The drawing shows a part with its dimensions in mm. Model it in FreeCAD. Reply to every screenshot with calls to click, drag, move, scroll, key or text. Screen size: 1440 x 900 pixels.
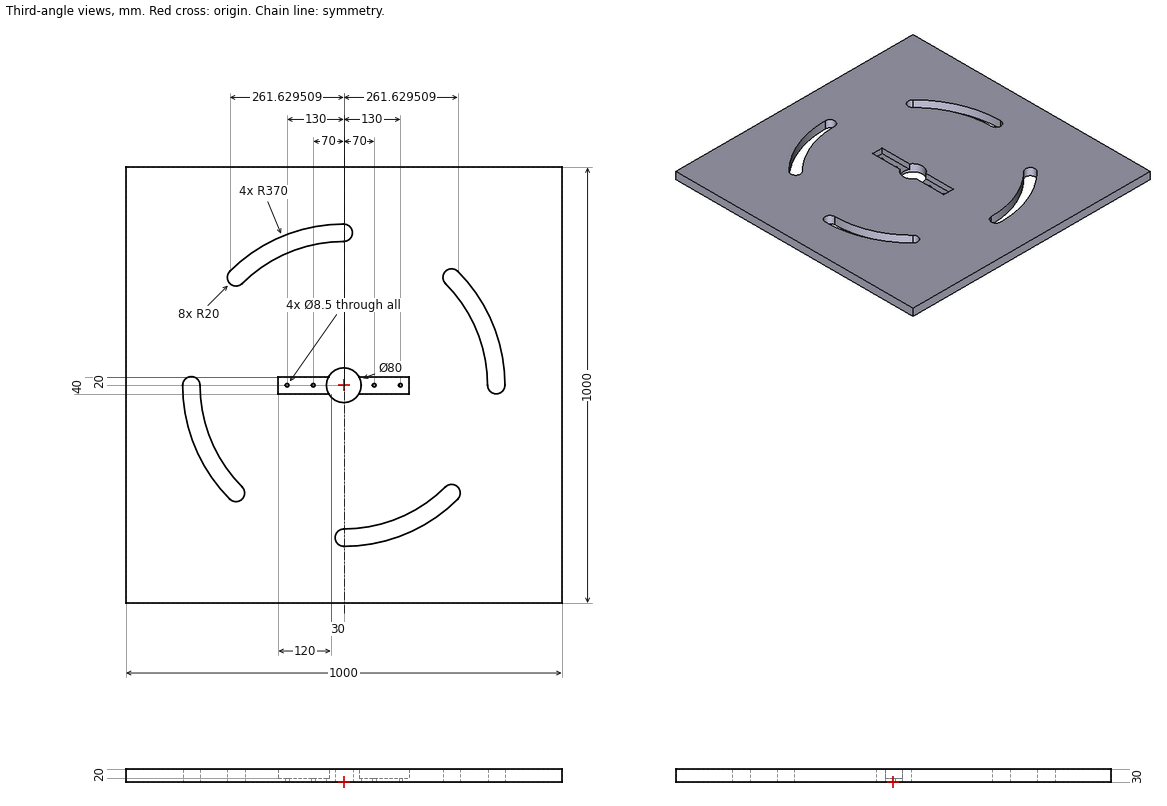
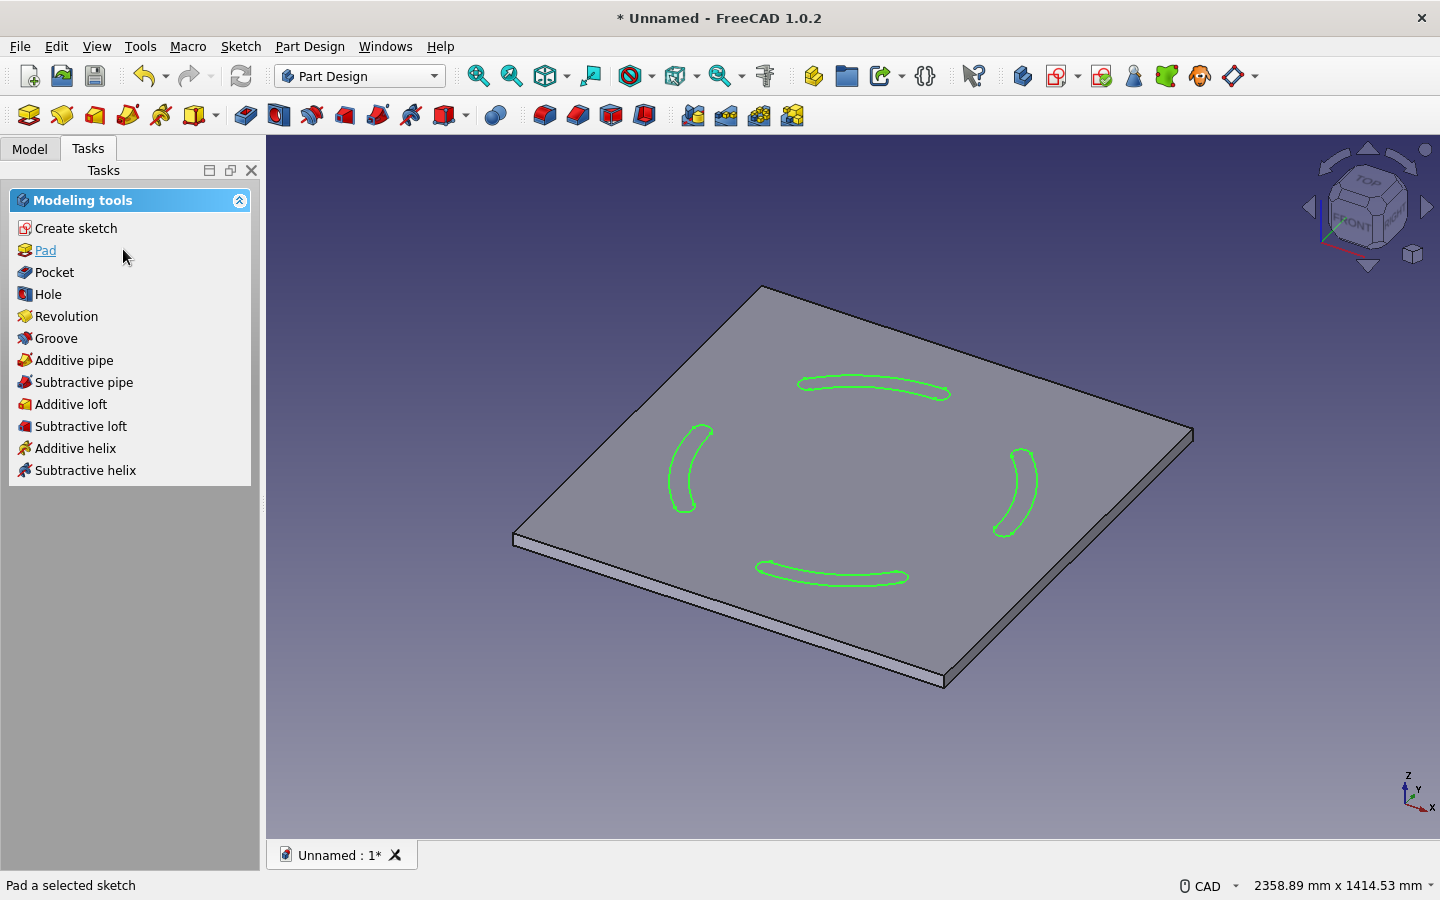
click(246, 116)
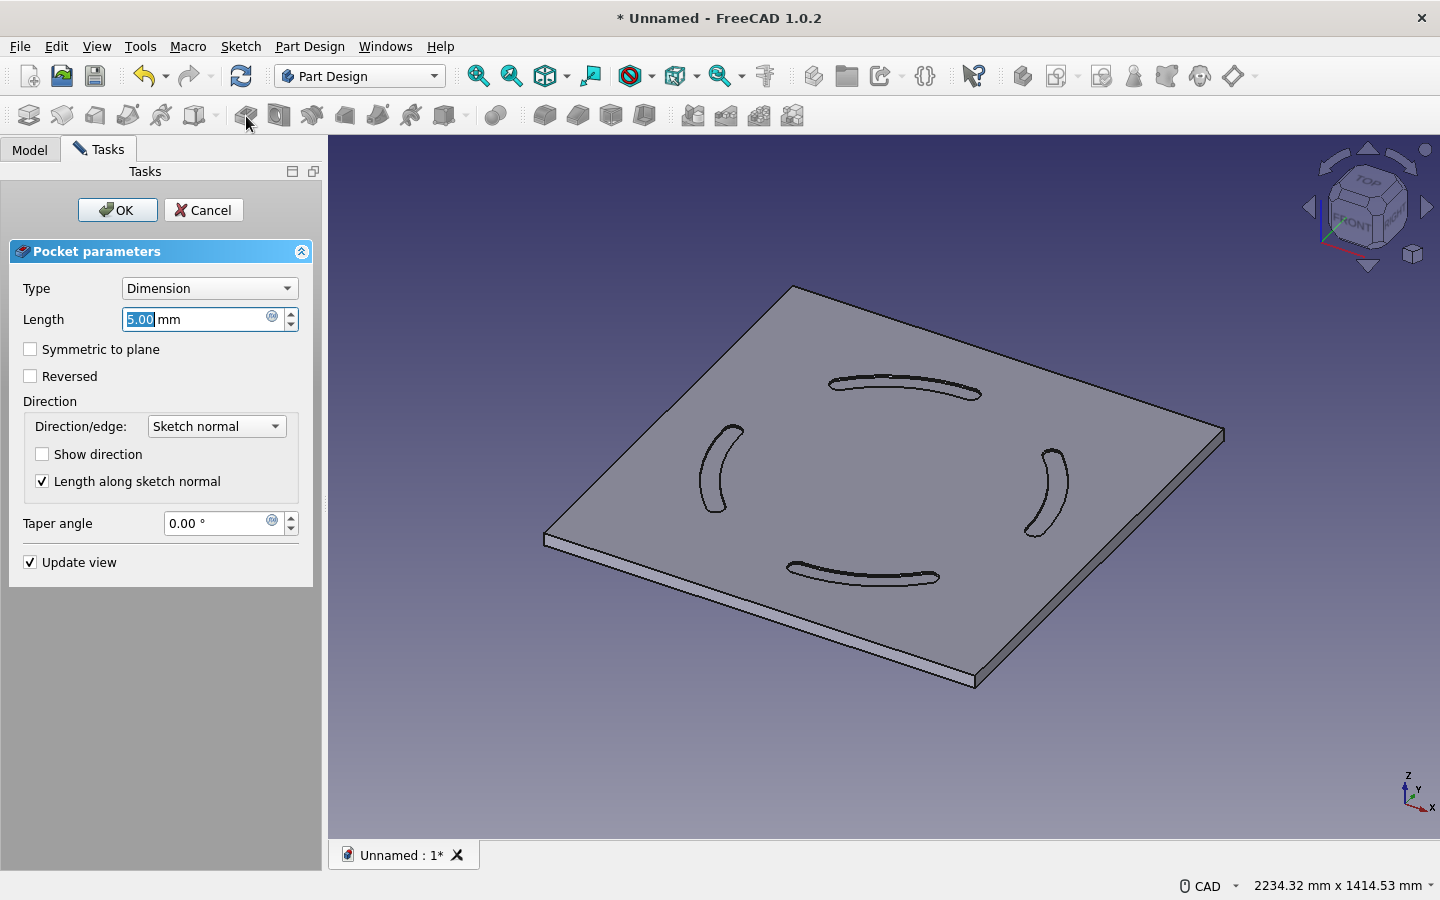
click(210, 288)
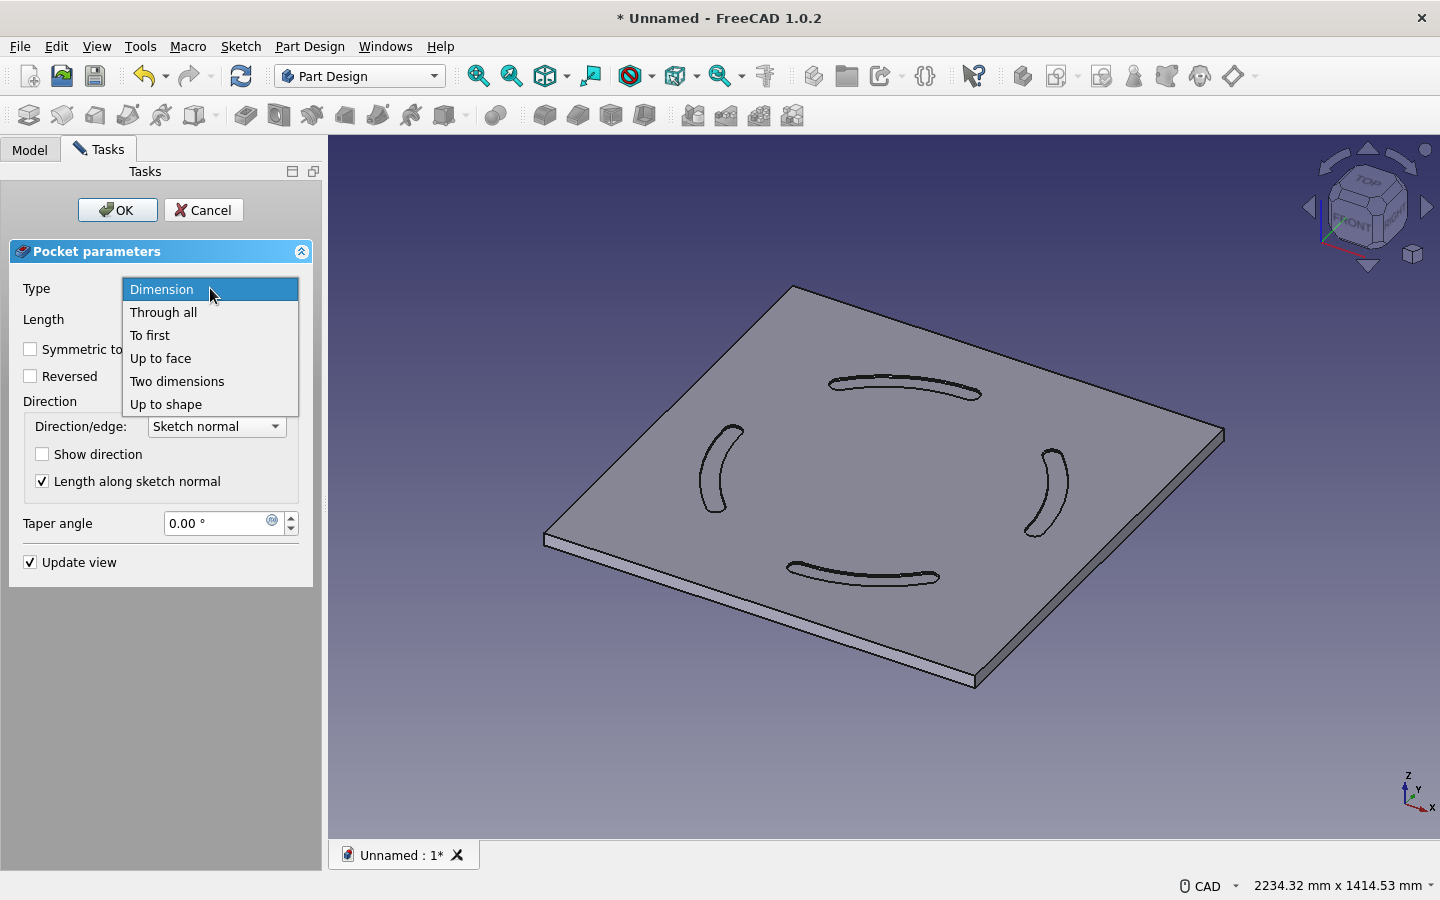
click(208, 312)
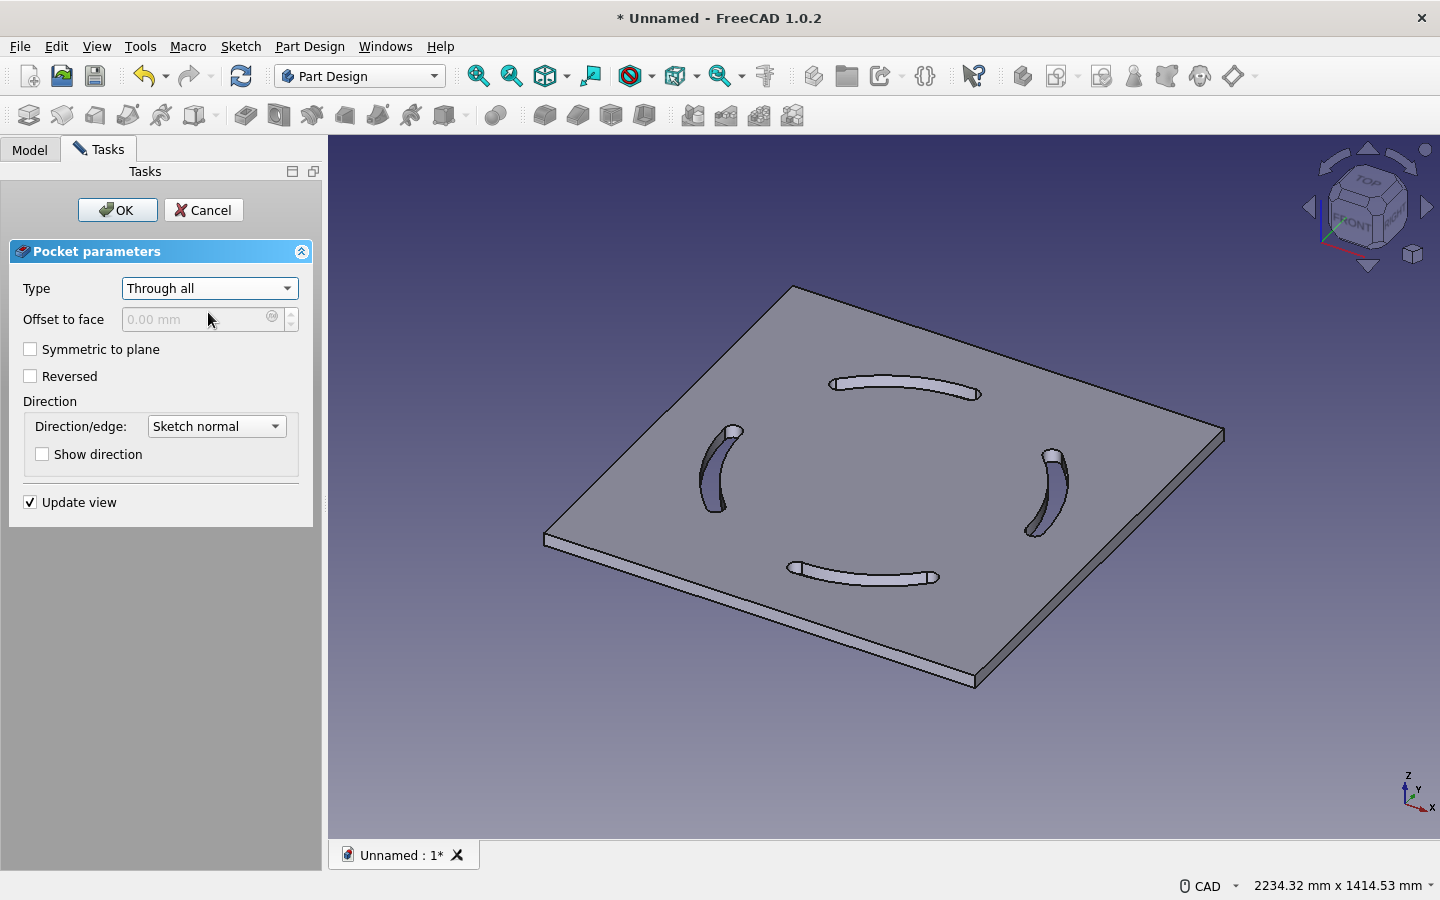
click(118, 210)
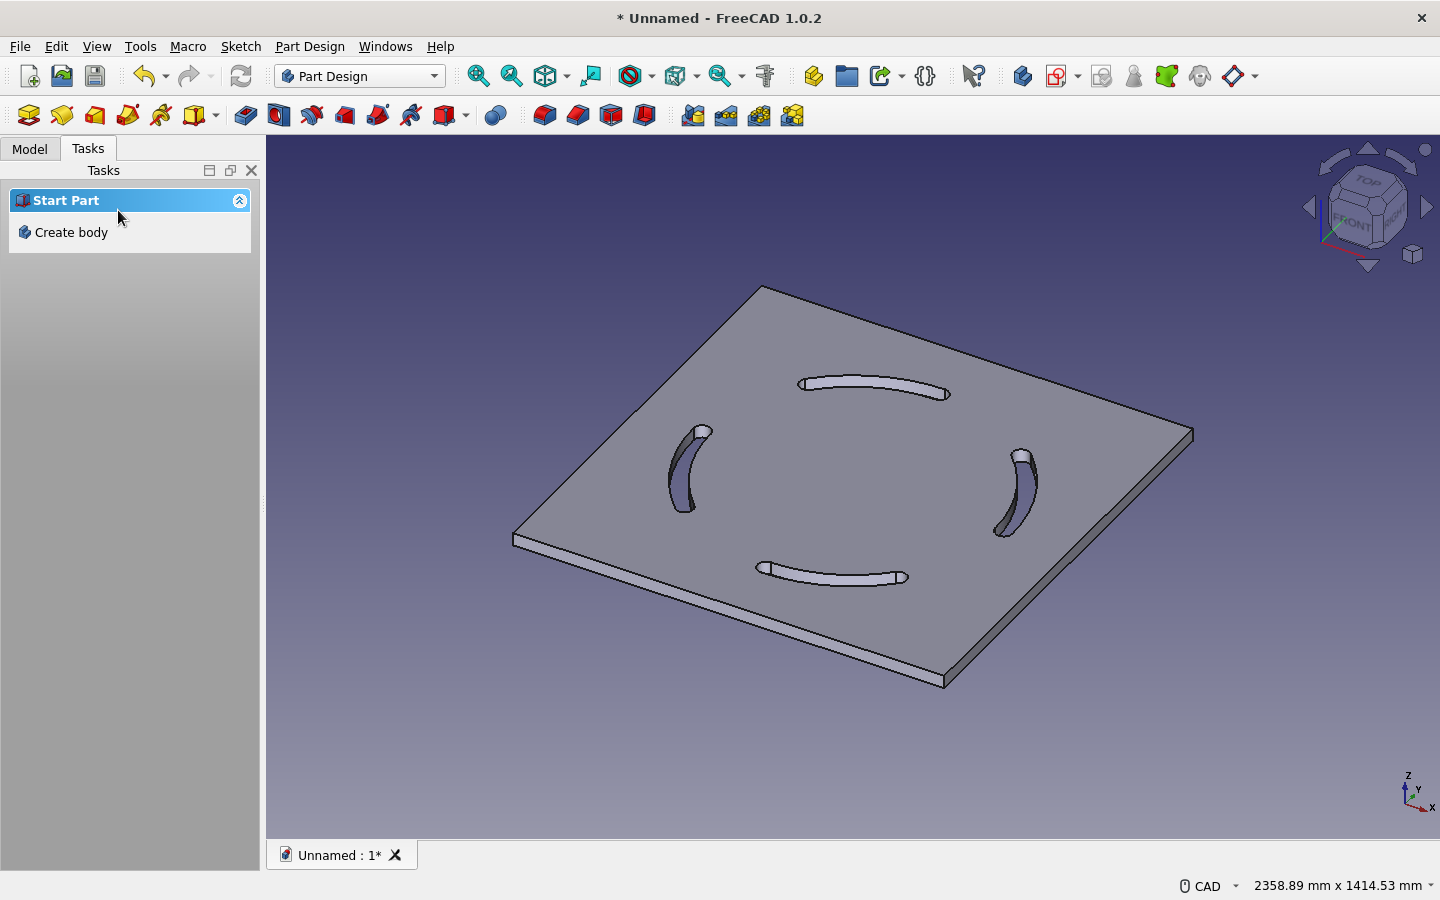
click(853, 480)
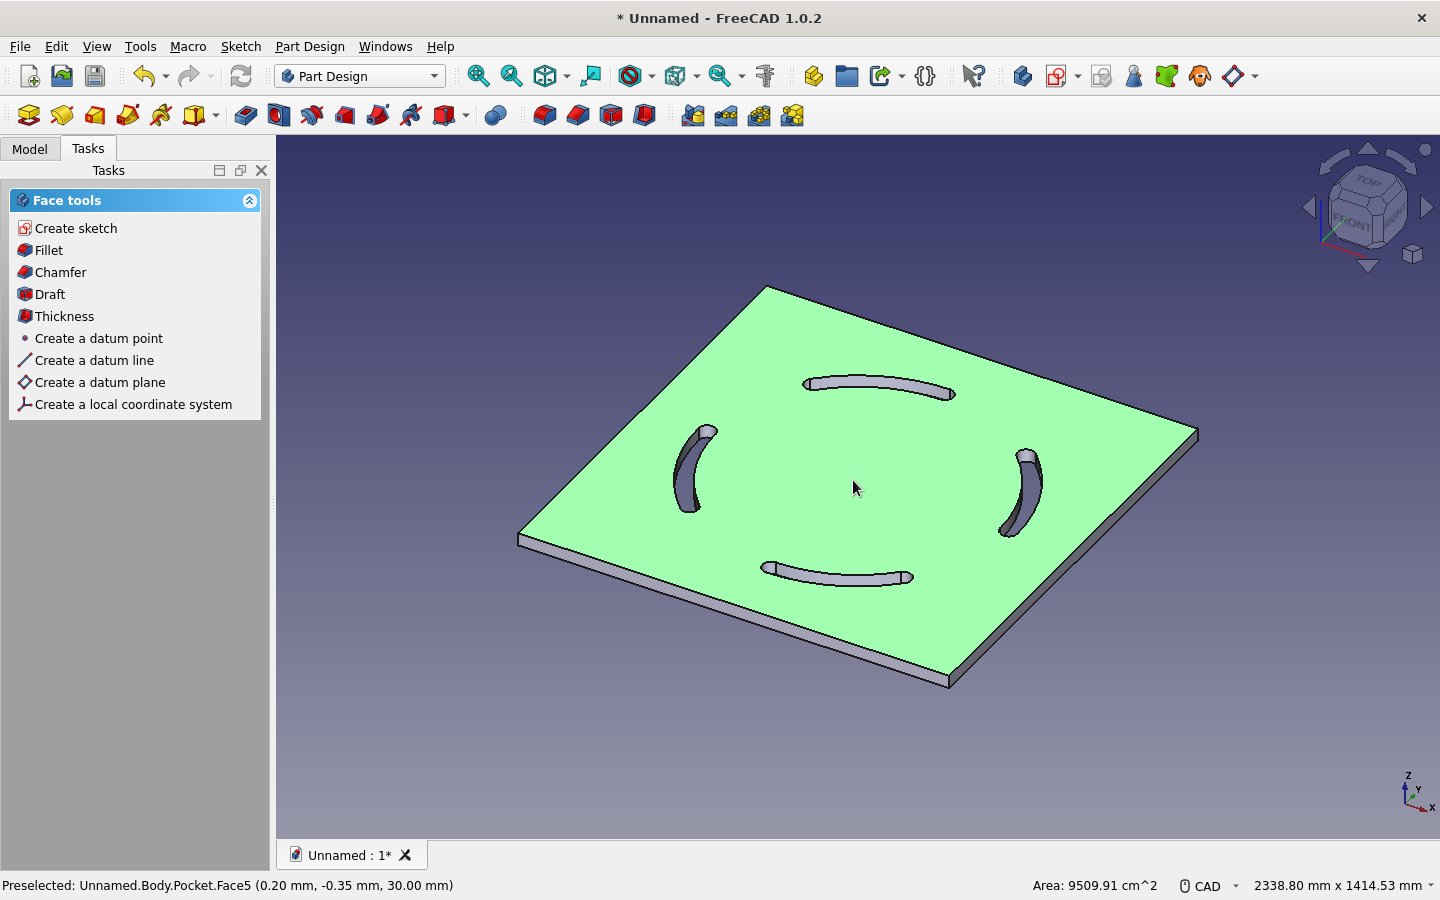
click(1056, 76)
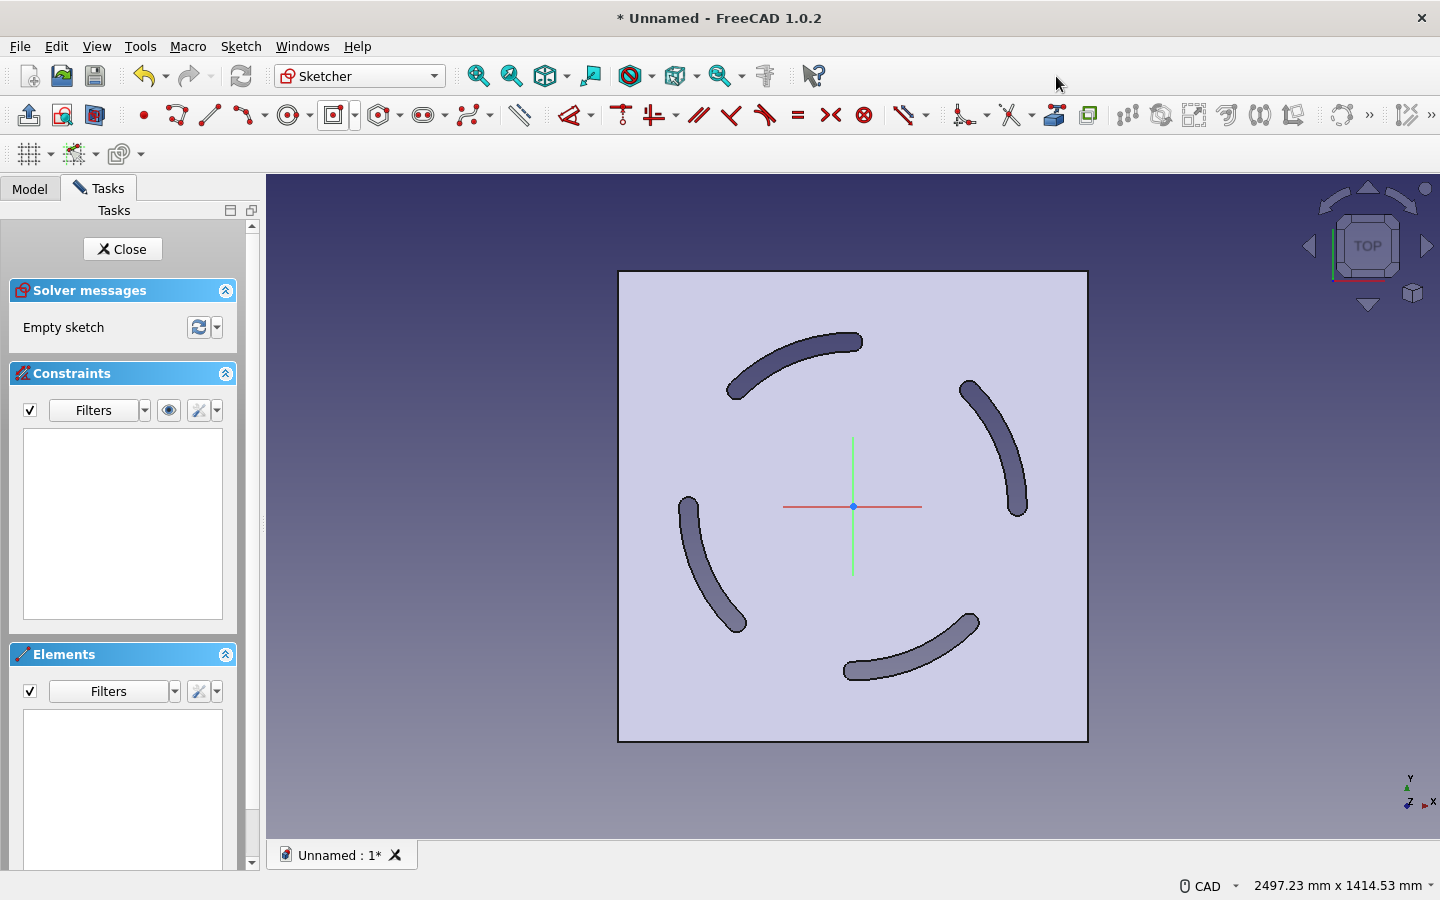
scroll(860, 506, up, 12)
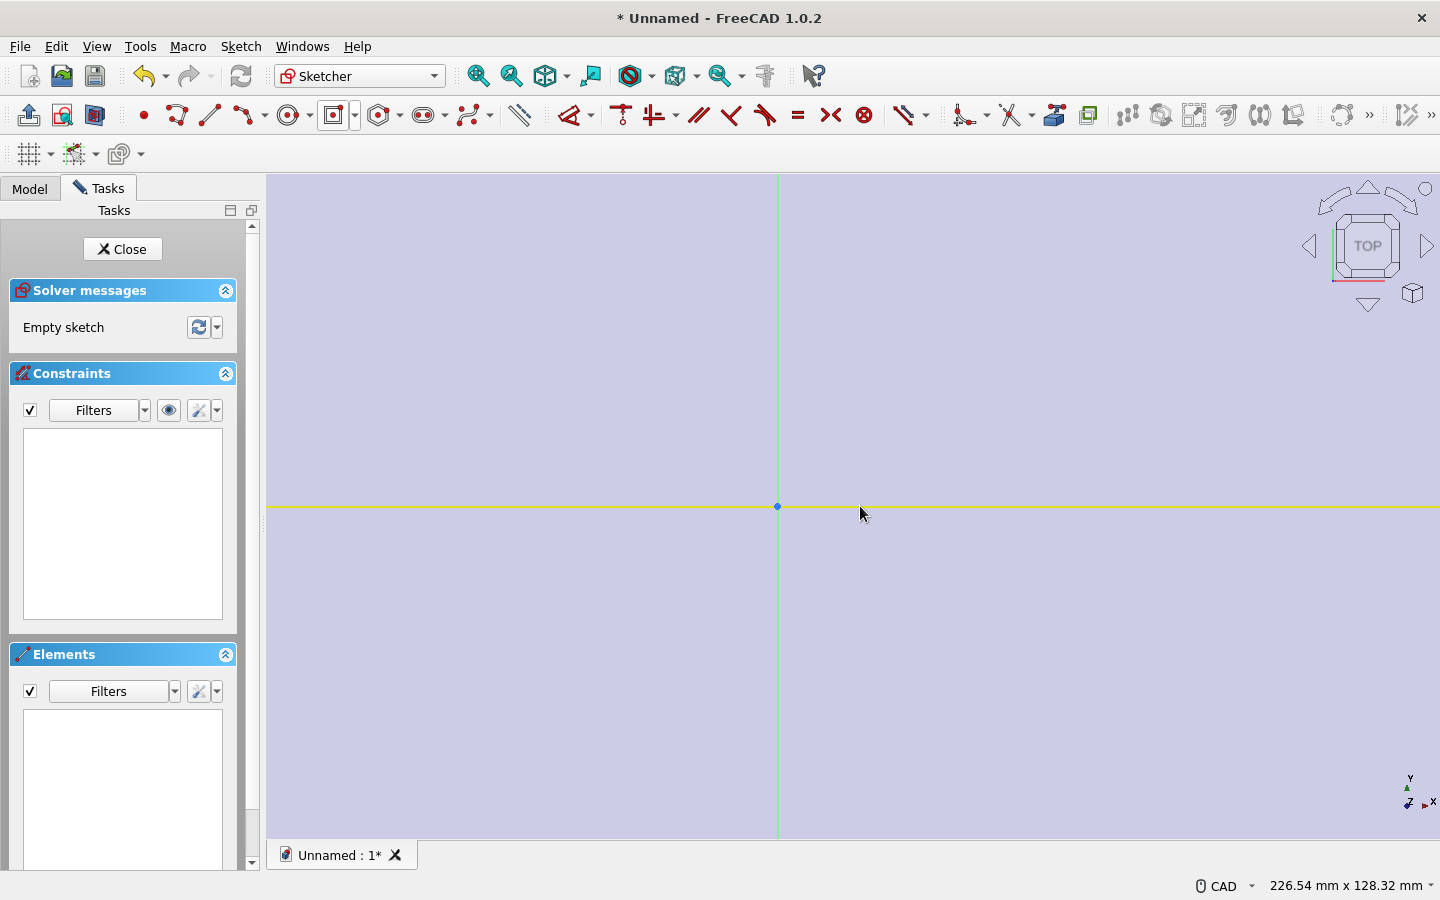
click(288, 116)